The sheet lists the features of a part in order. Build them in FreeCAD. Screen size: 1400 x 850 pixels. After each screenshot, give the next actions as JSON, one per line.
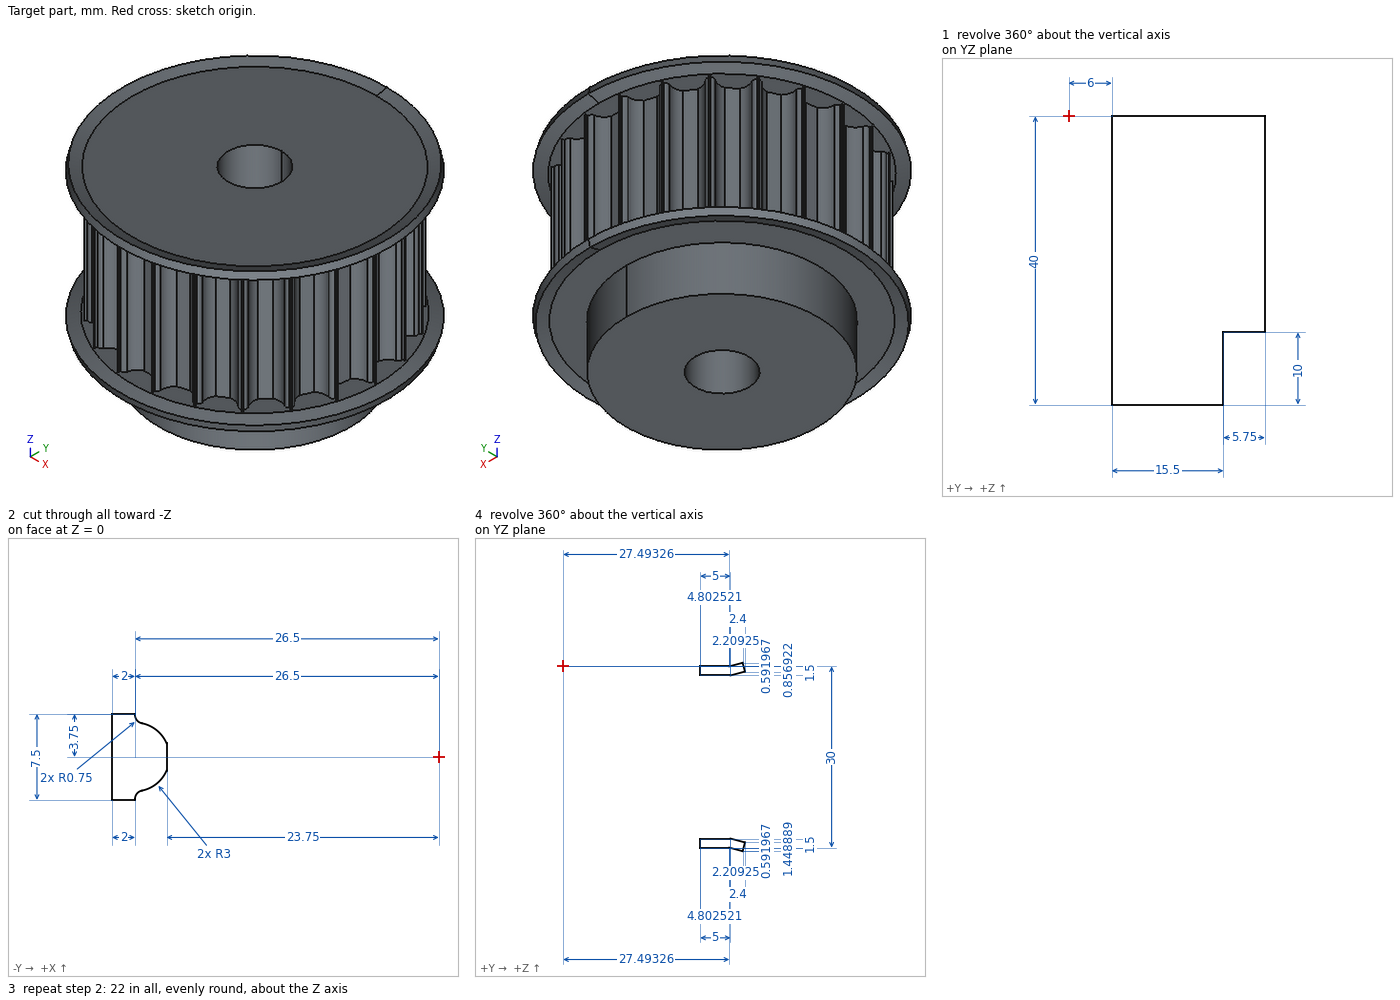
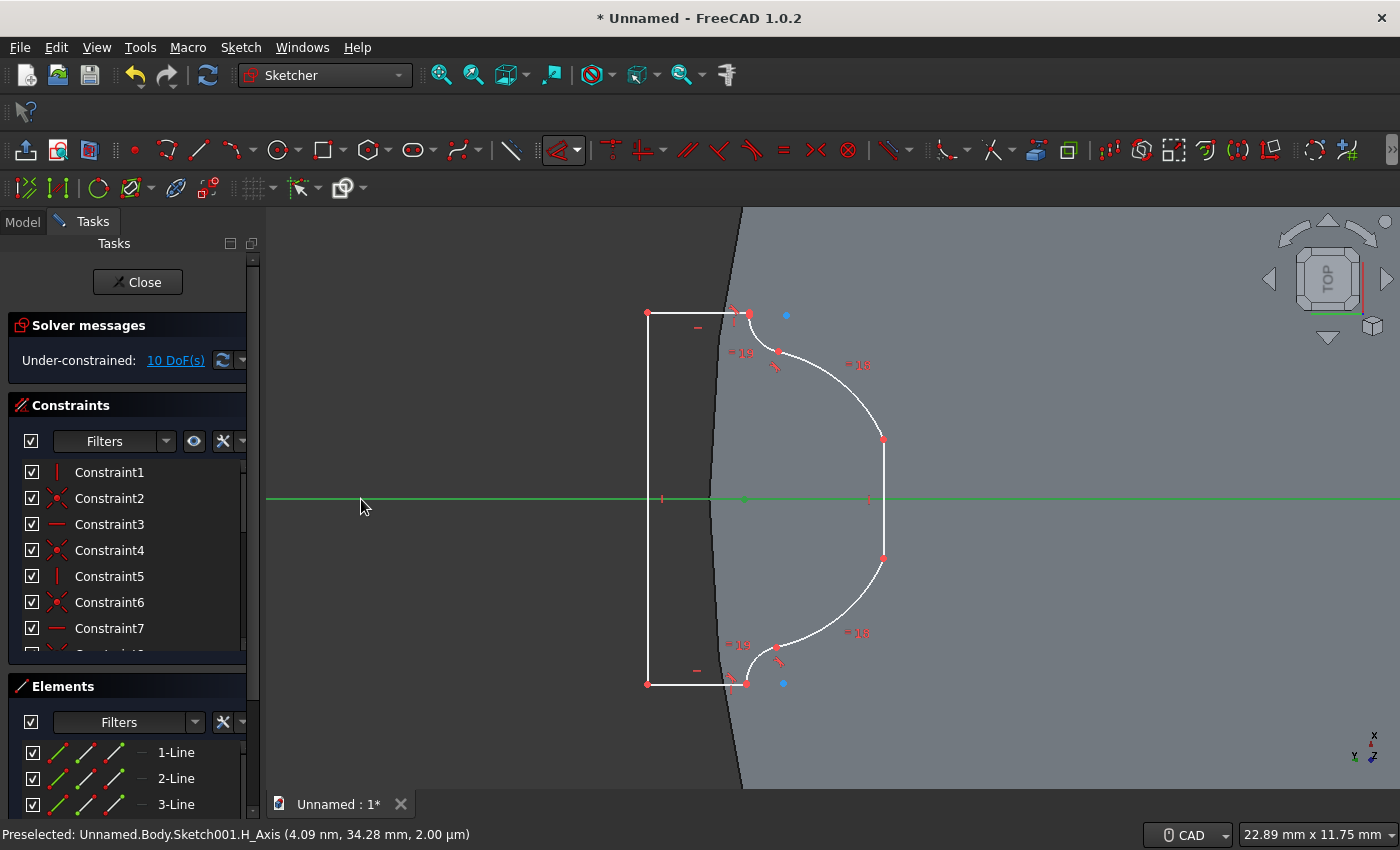
{"action": "left_click", "coordinate": [612, 150]}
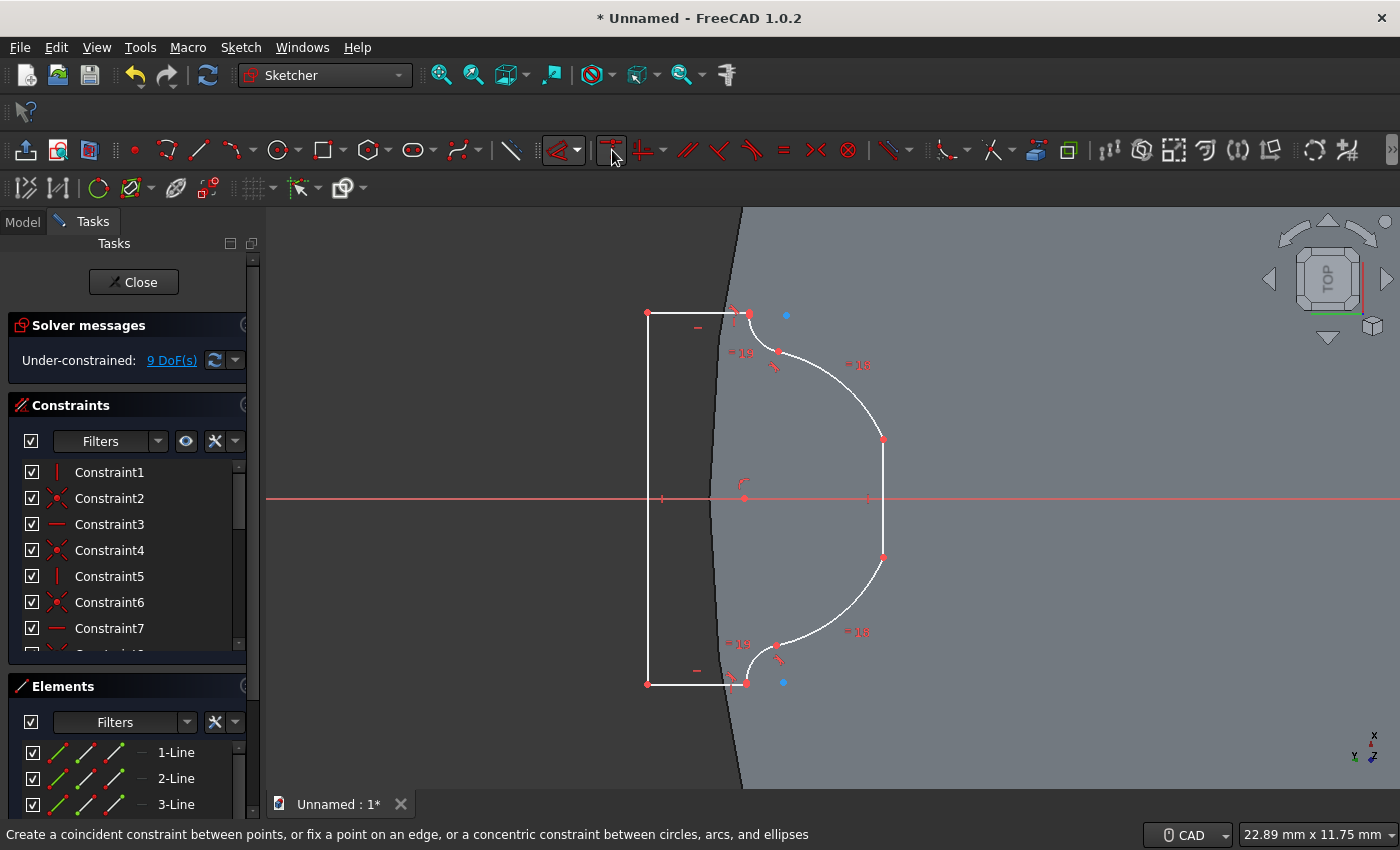
{"action": "left_click", "coordinate": [762, 652]}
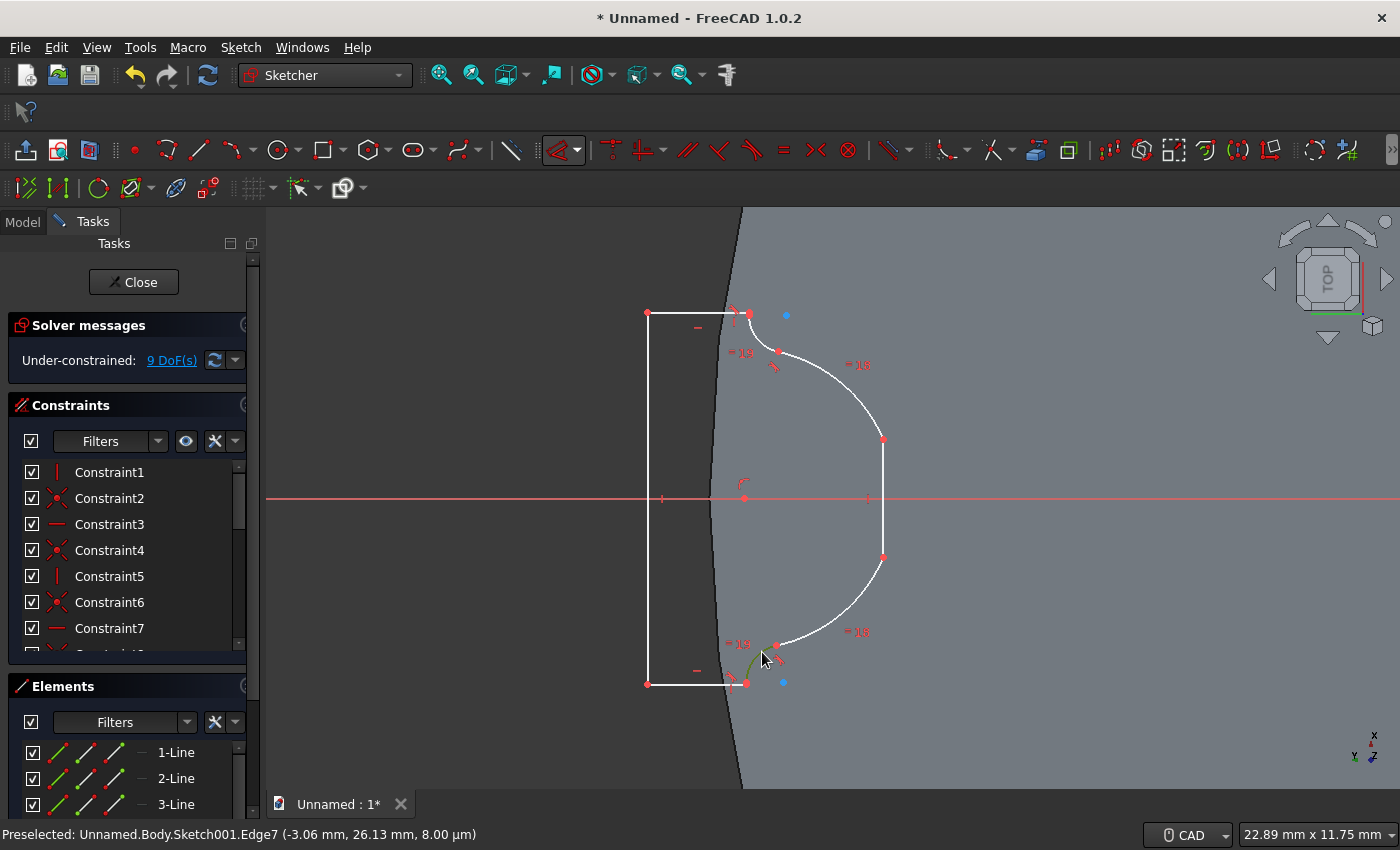
{"action": "left_click", "coordinate": [580, 150]}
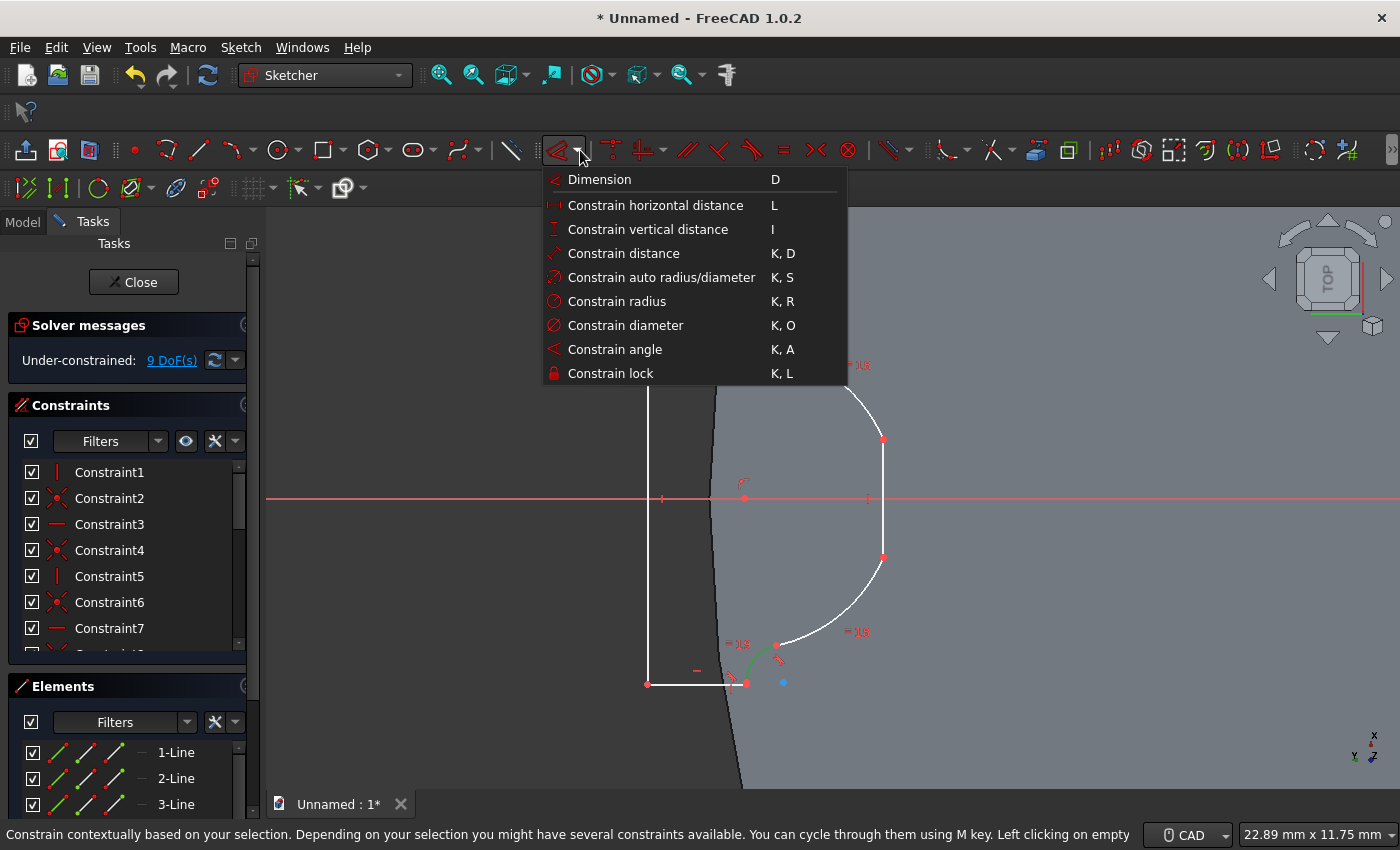
{"action": "left_click", "coordinate": [695, 301]}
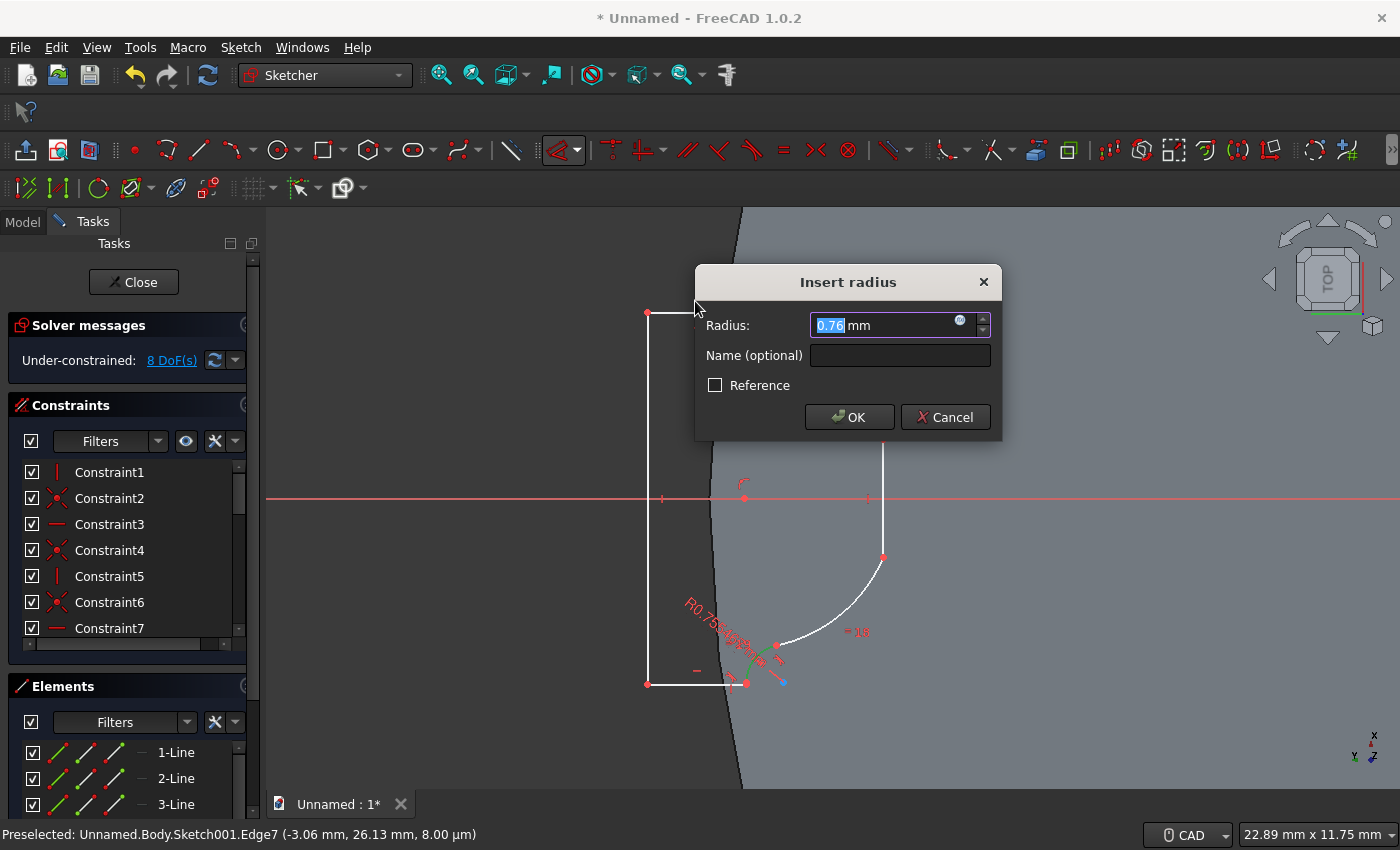
{"action": "type", "text": "0.75"}
{"action": "key", "text": "Return"}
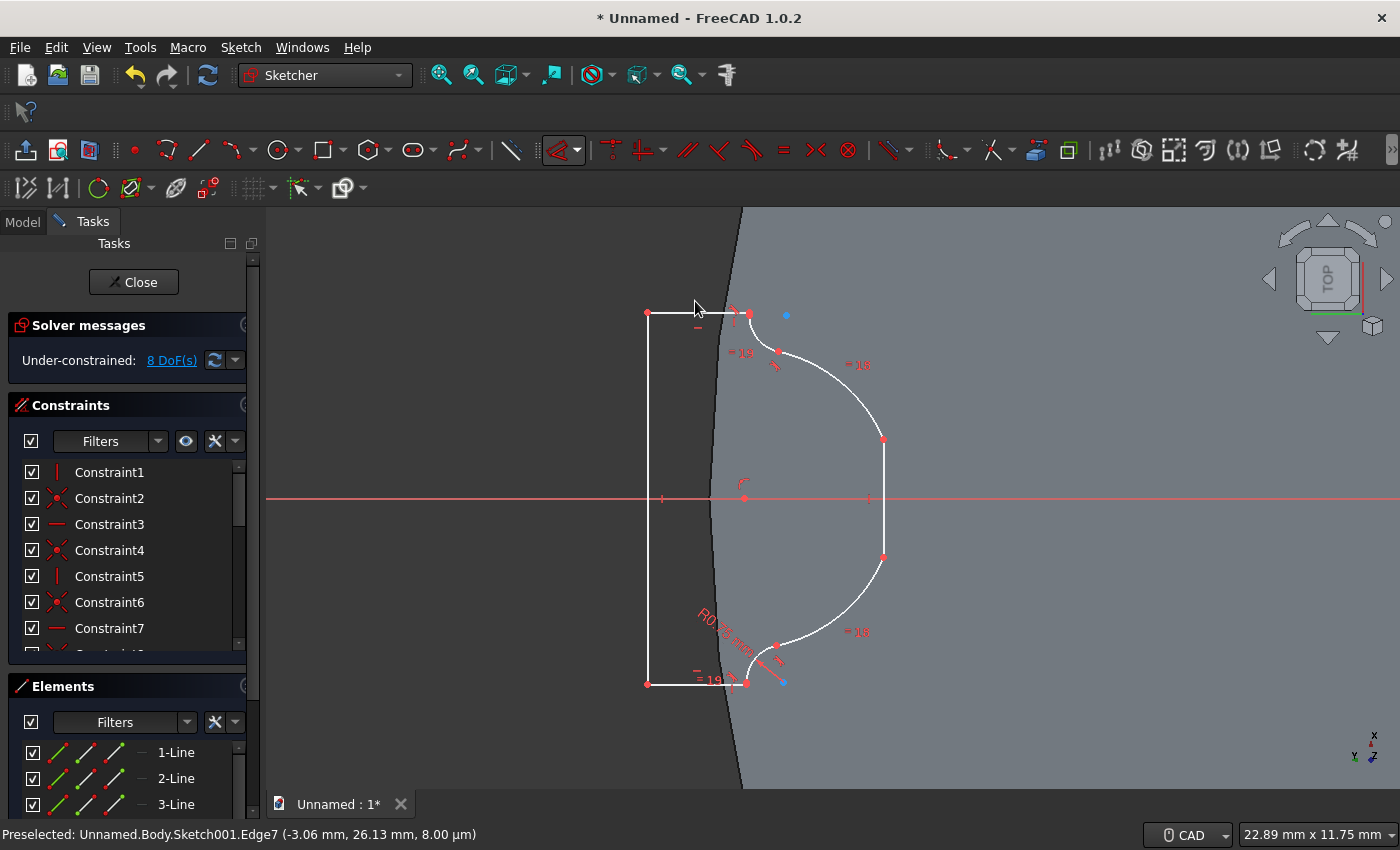
{"action": "left_click", "coordinate": [817, 631]}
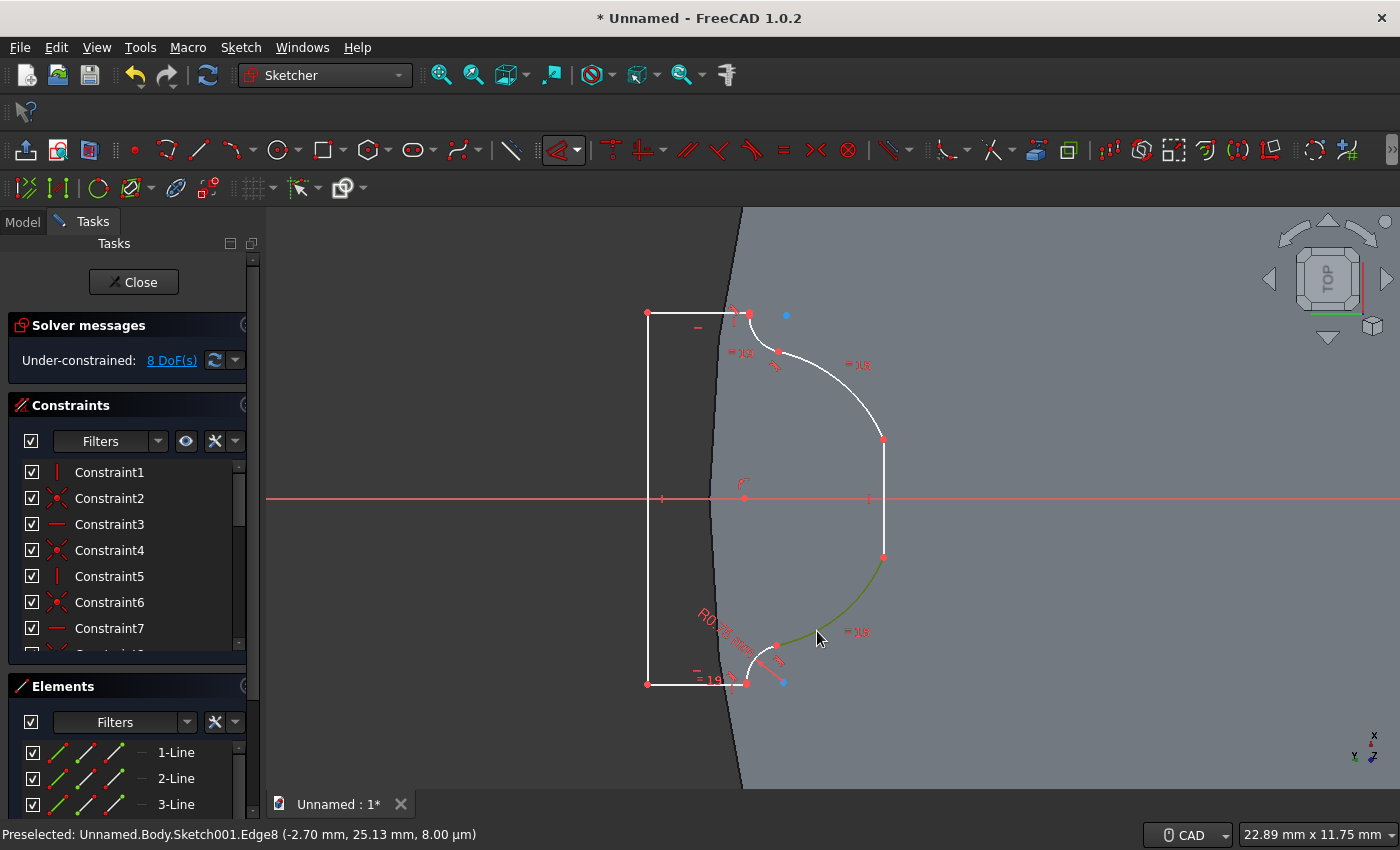
{"action": "key", "text": "k r"}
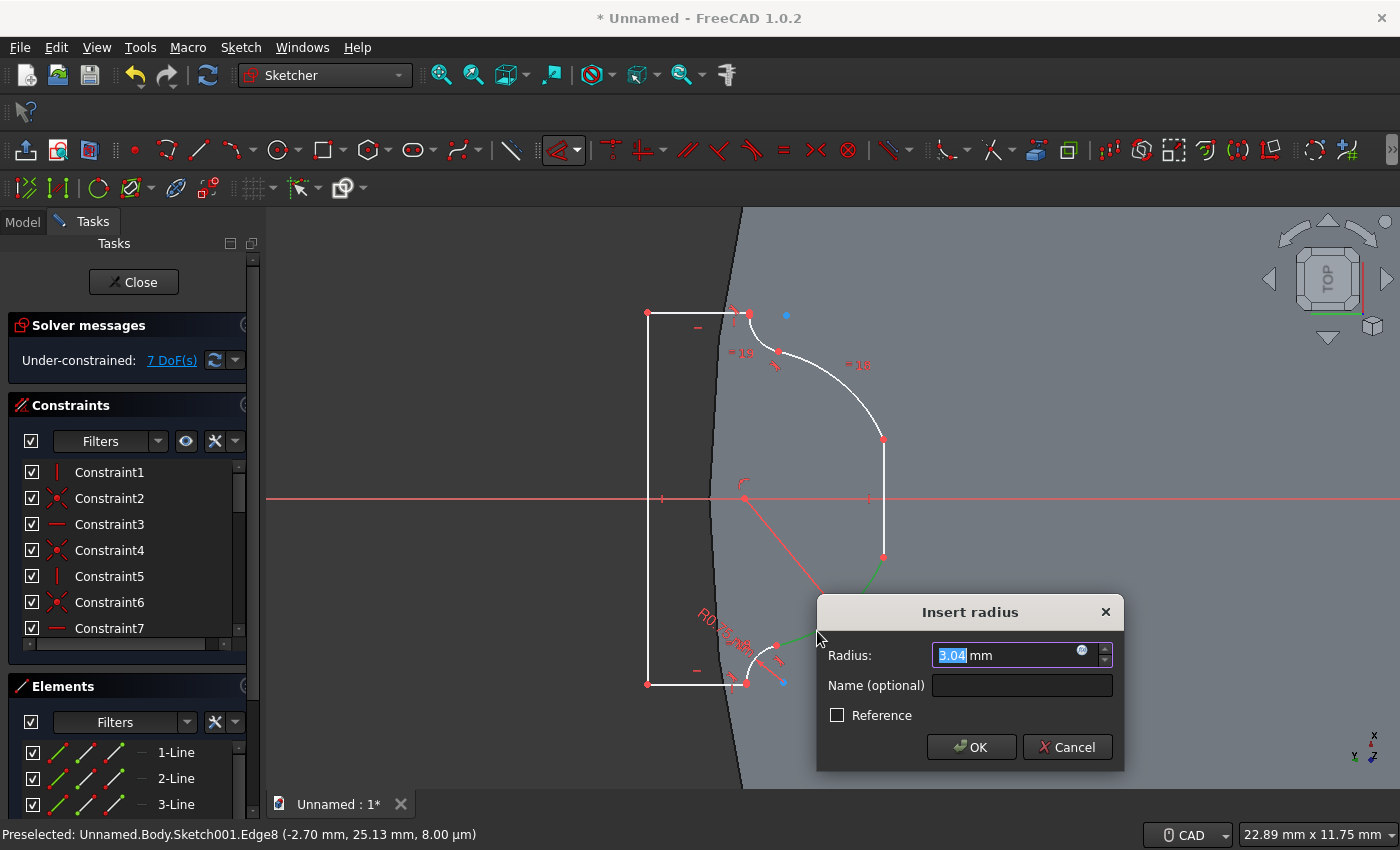
{"action": "type", "text": "3"}
{"action": "key", "text": "Return"}